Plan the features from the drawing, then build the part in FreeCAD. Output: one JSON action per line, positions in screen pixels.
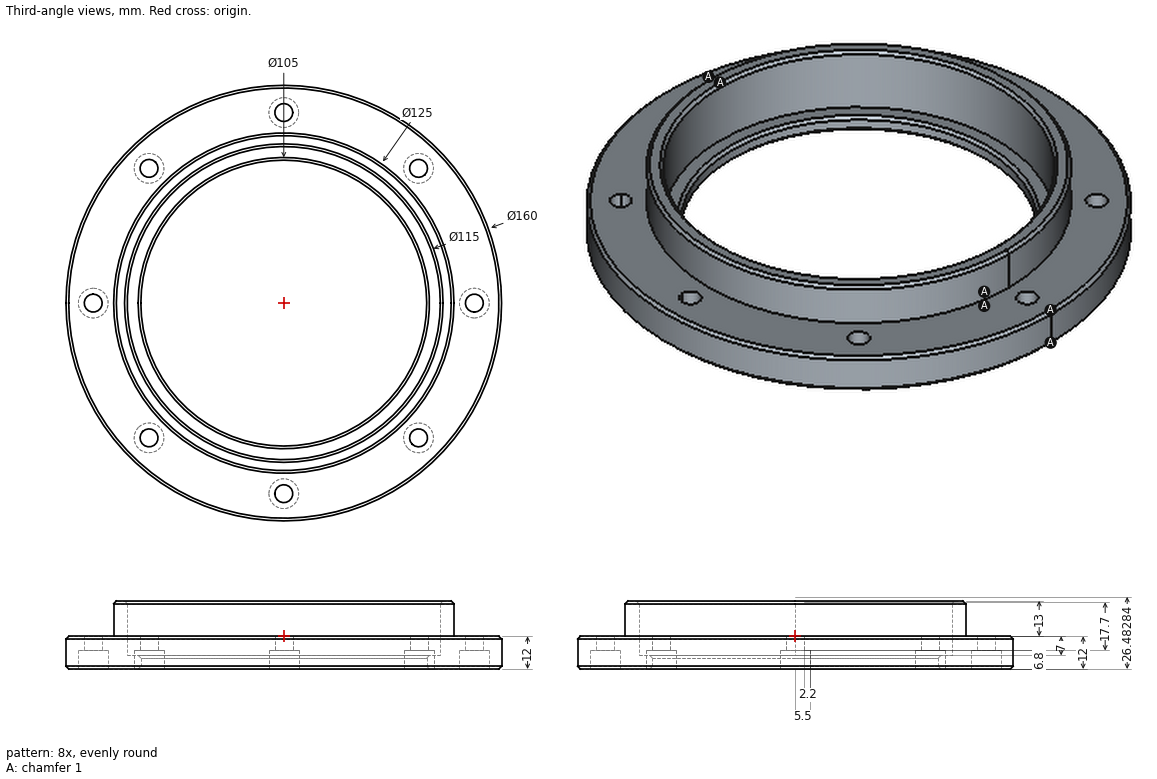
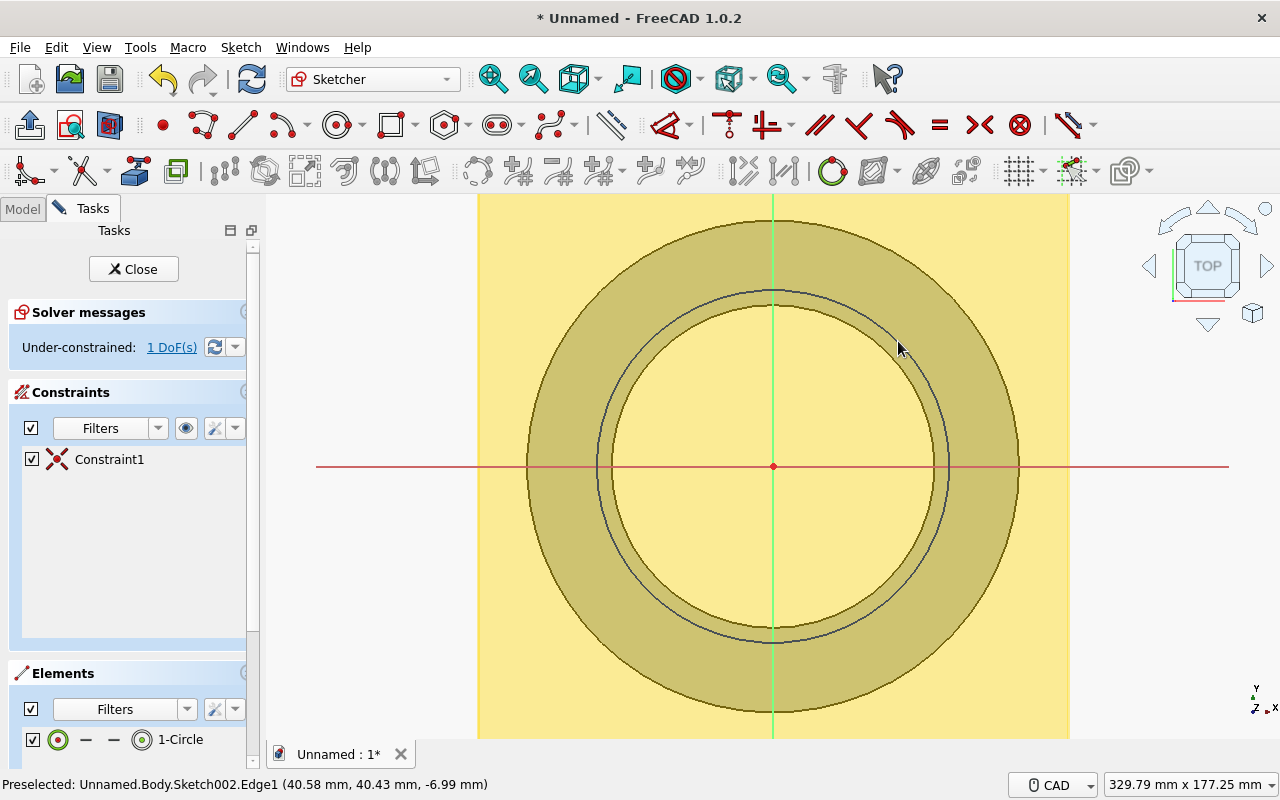
{"action": "left_click", "coordinate": [897, 341]}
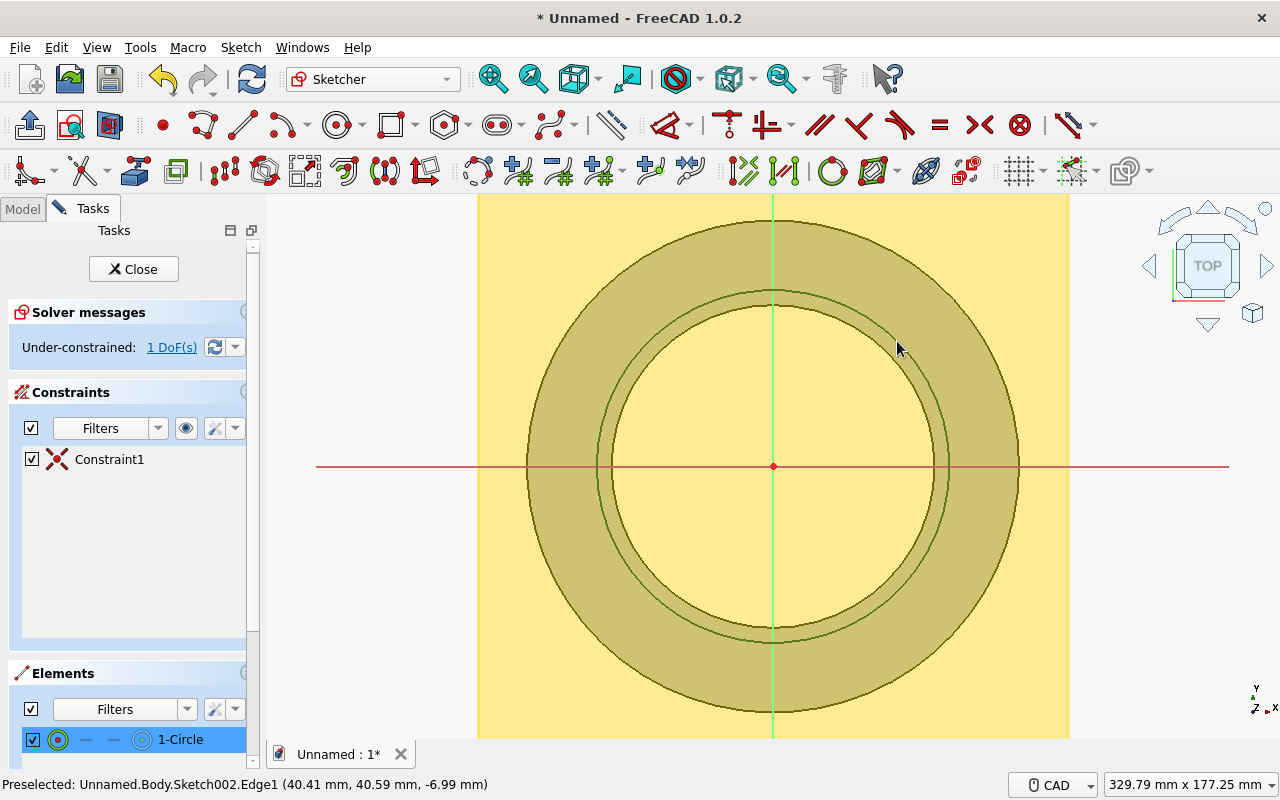
{"action": "key", "text": "k o"}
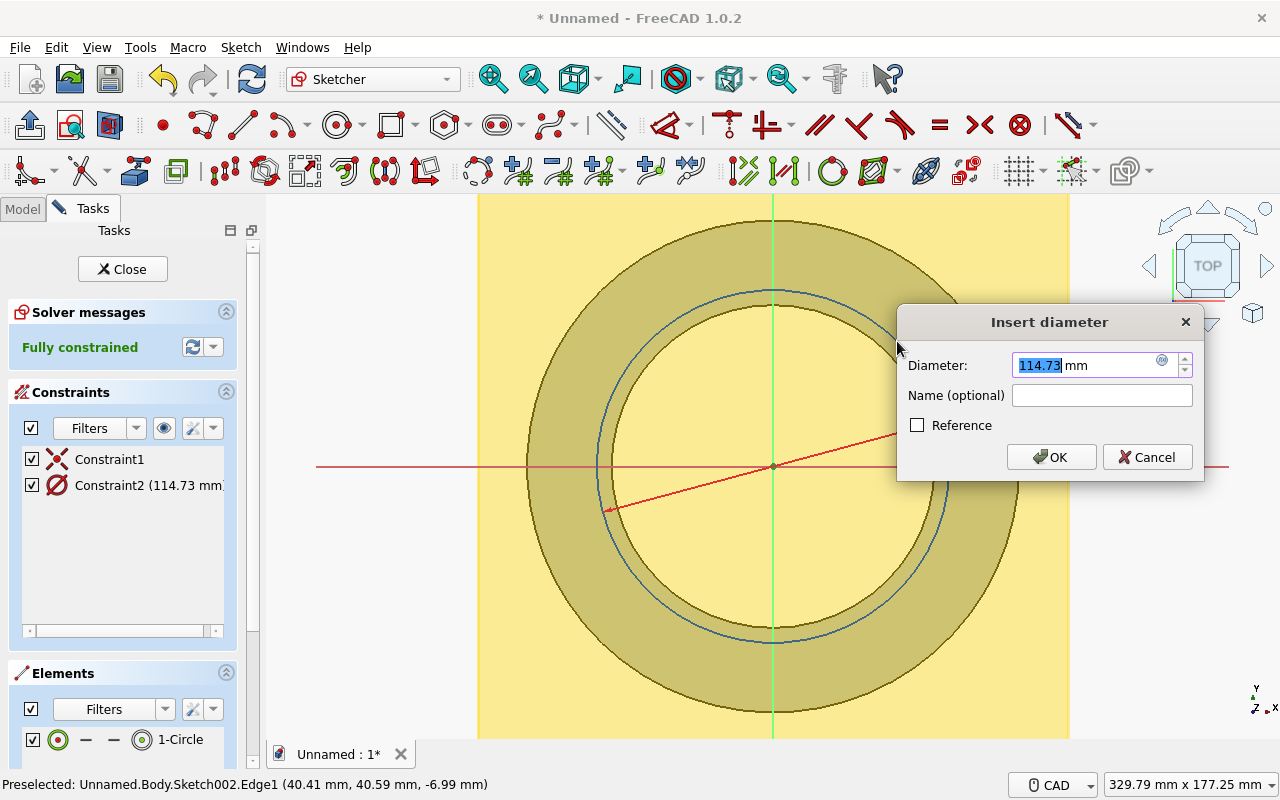
{"action": "type", "text": "115"}
{"action": "key", "text": "Return"}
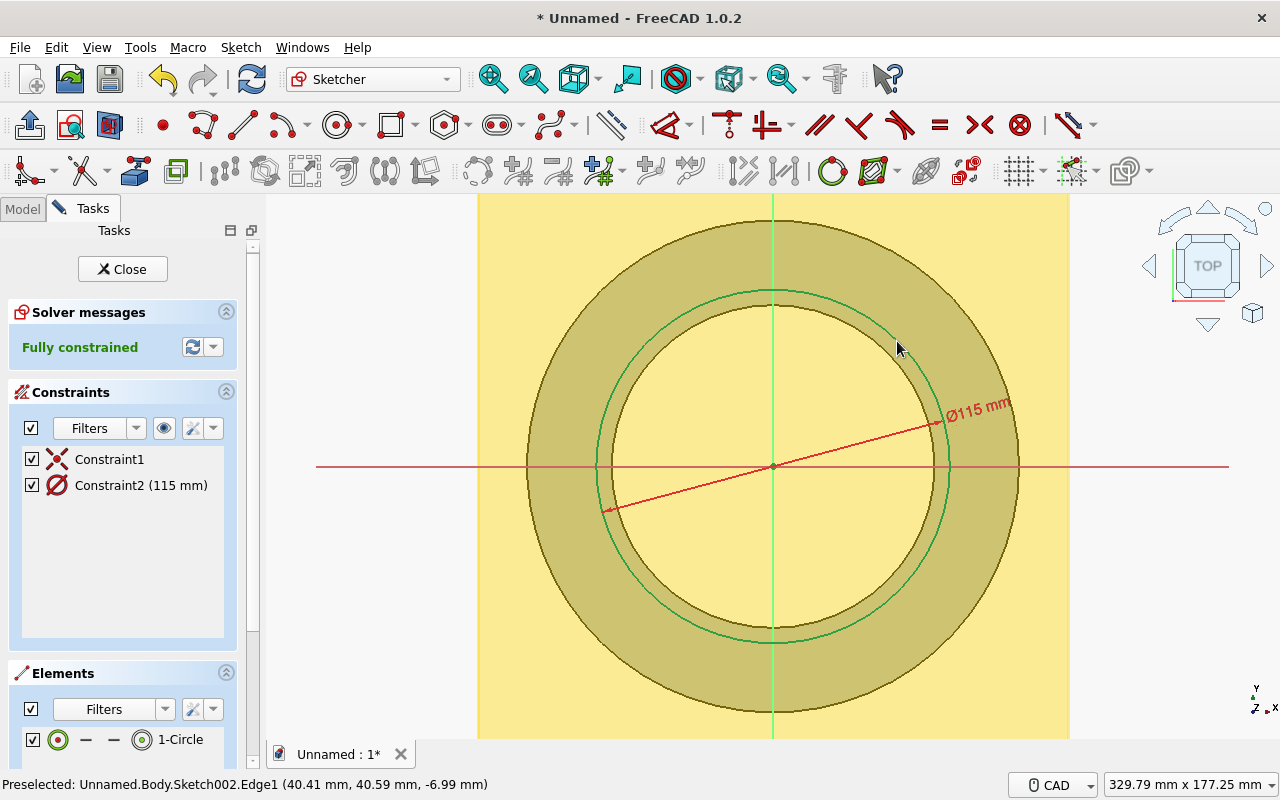
{"action": "left_click", "coordinate": [123, 269]}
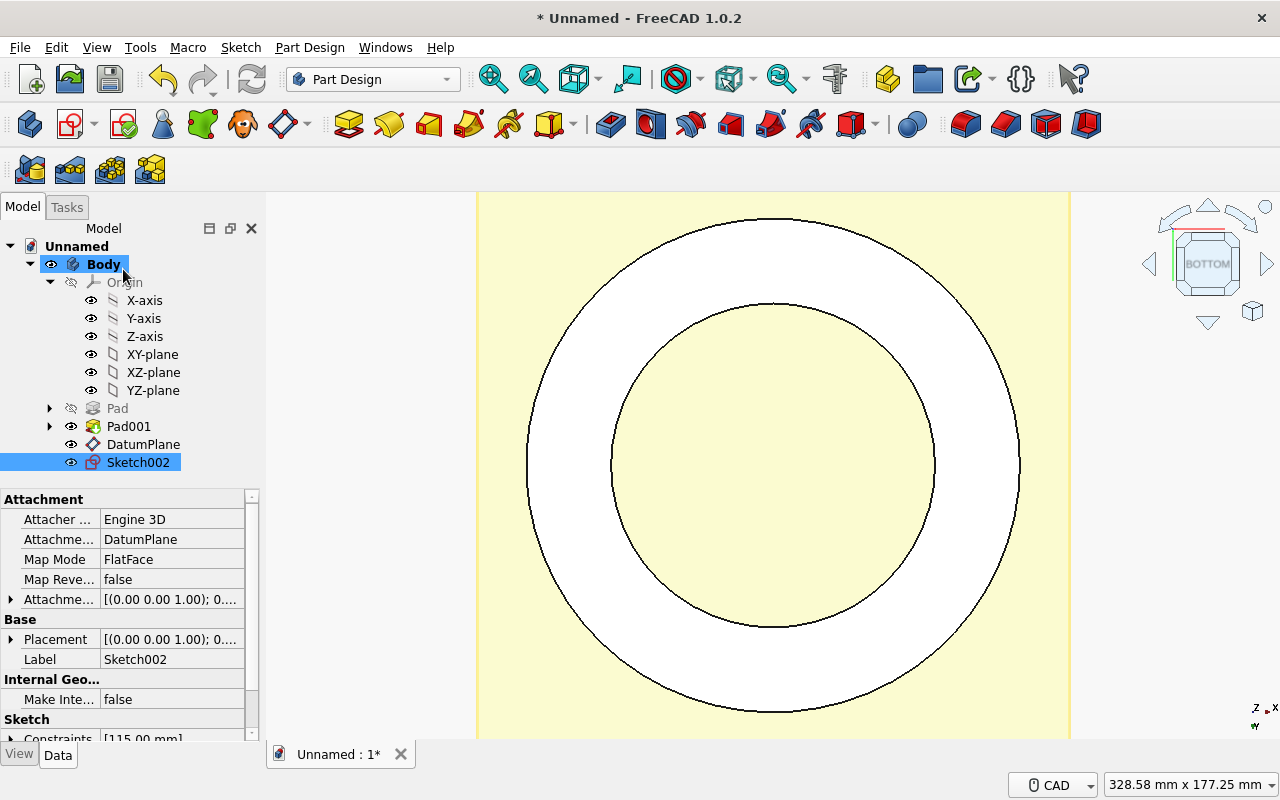
{"action": "left_click", "coordinate": [612, 124]}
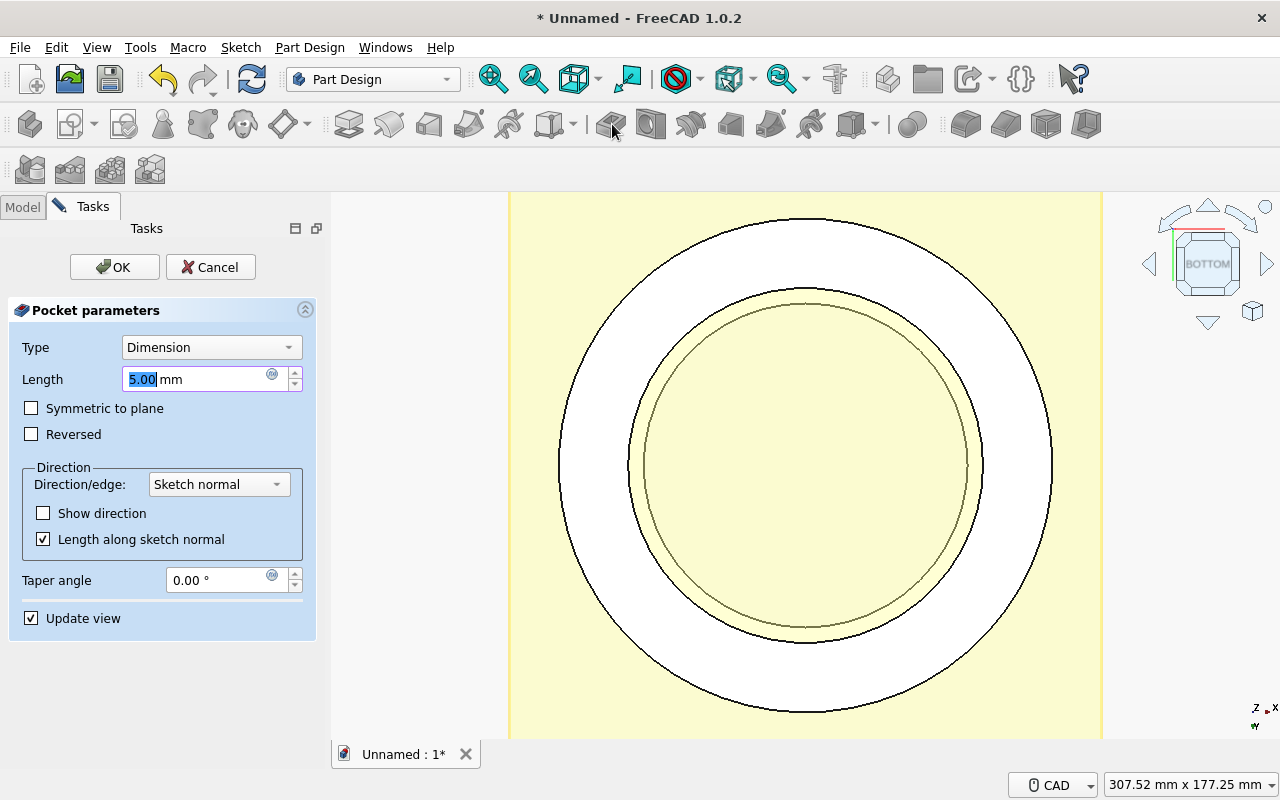
{"action": "type", "text": "7"}
{"action": "key", "text": "Tab"}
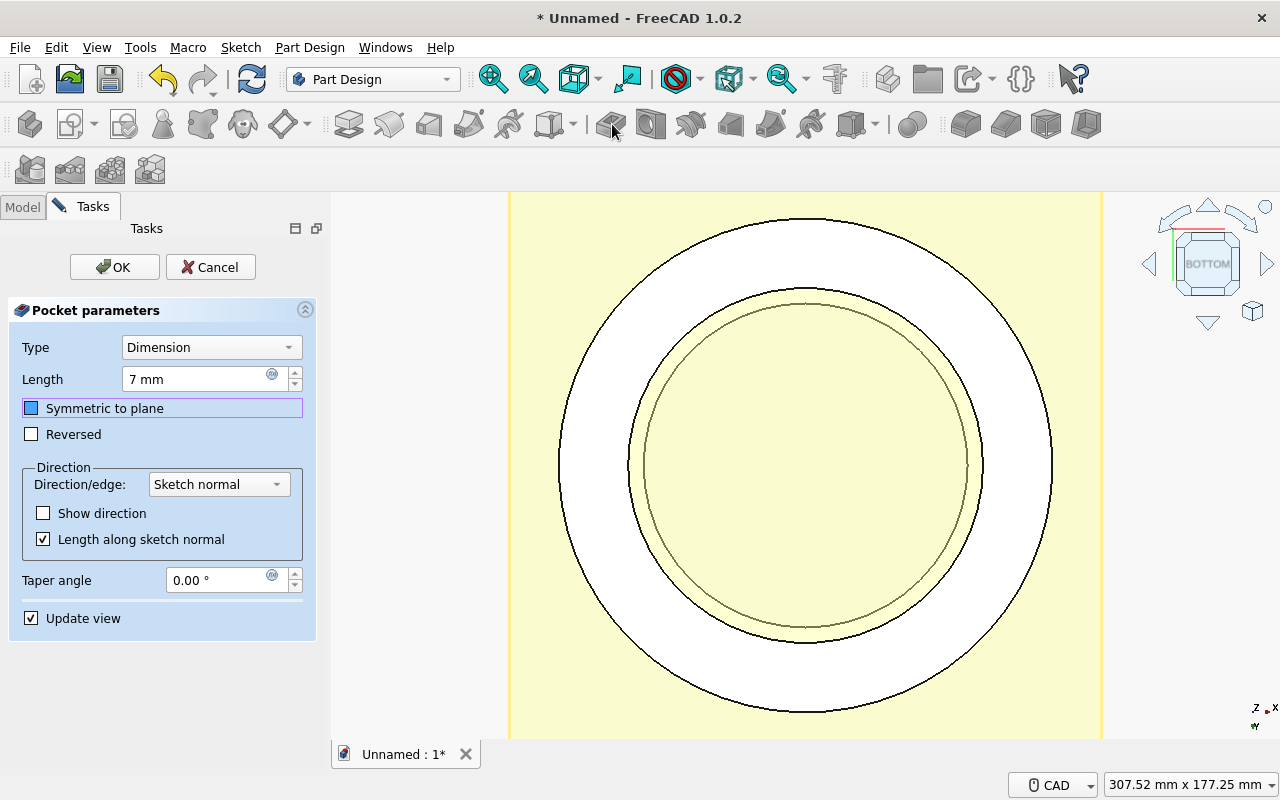
{"action": "left_click", "coordinate": [30, 434]}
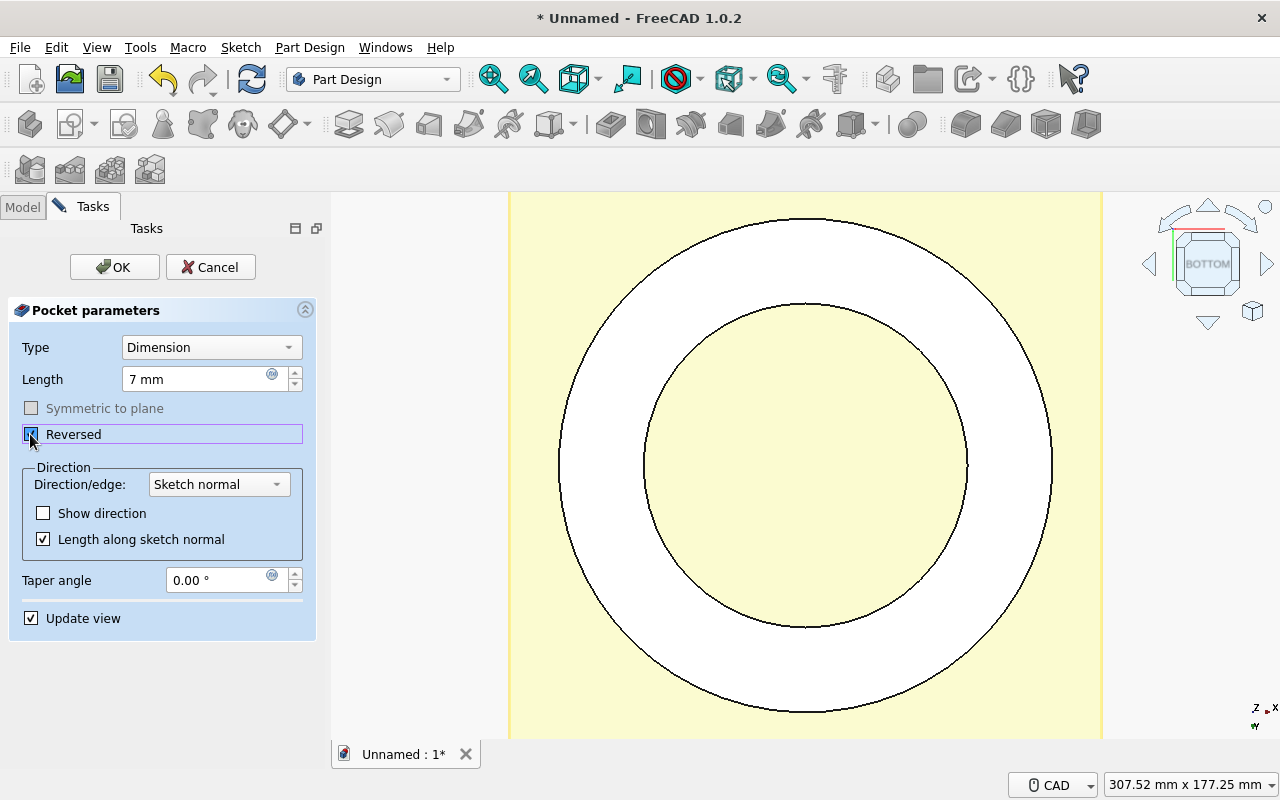
{"action": "left_click", "coordinate": [115, 267]}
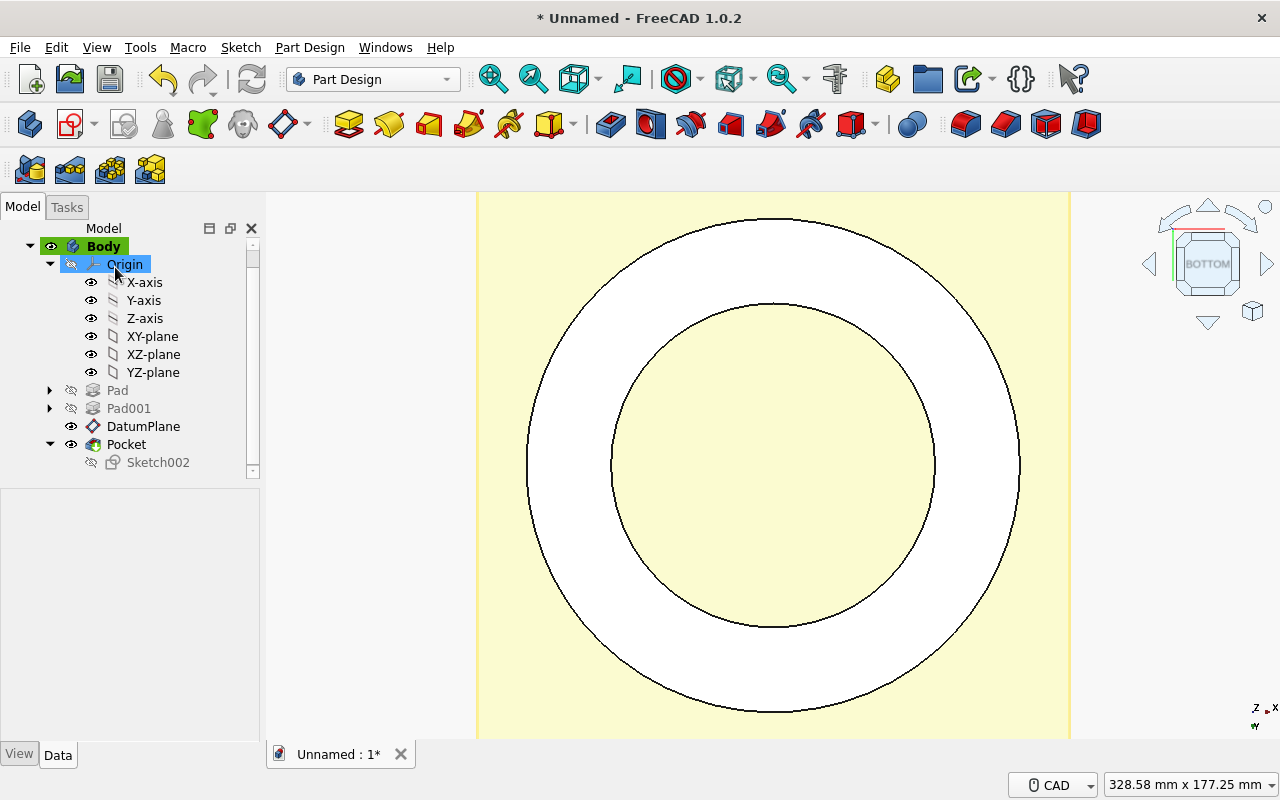
{"action": "left_click", "coordinate": [116, 426]}
{"action": "key", "text": "space"}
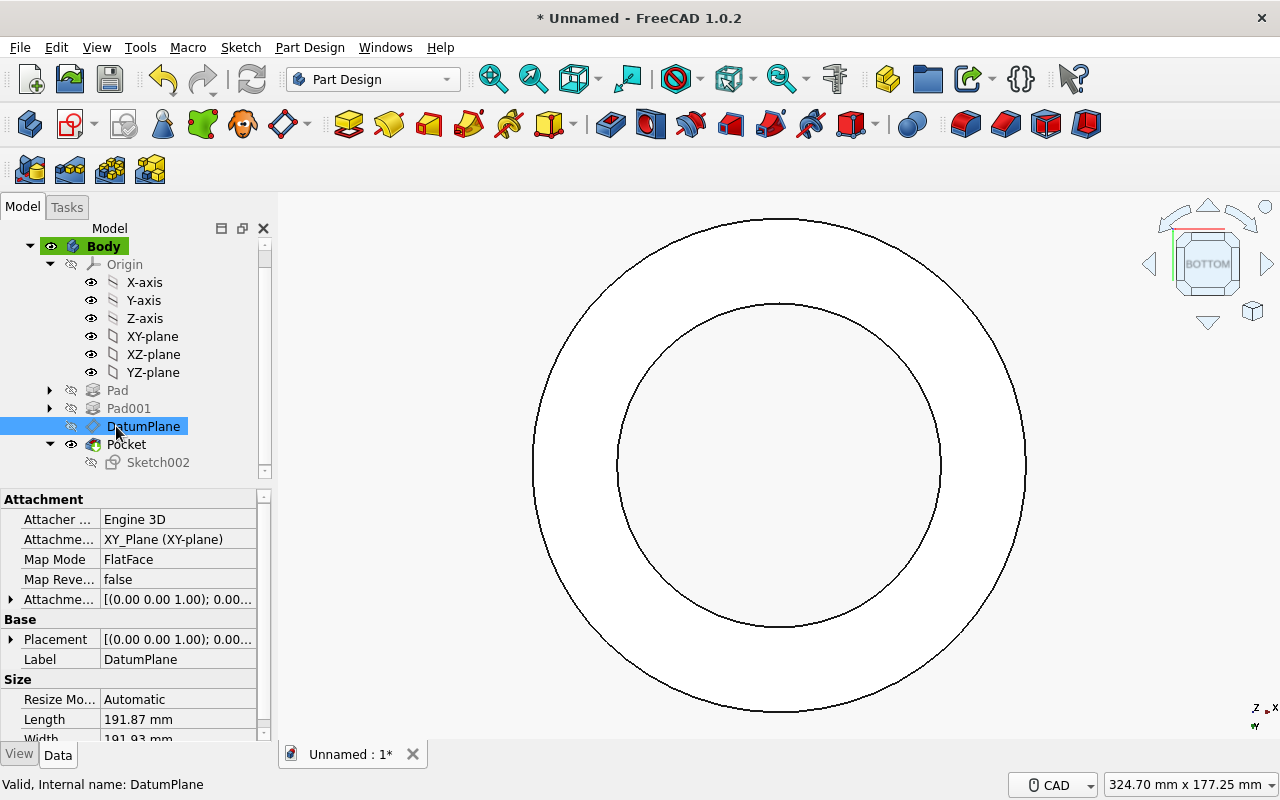
{"action": "left_click", "coordinate": [136, 372]}